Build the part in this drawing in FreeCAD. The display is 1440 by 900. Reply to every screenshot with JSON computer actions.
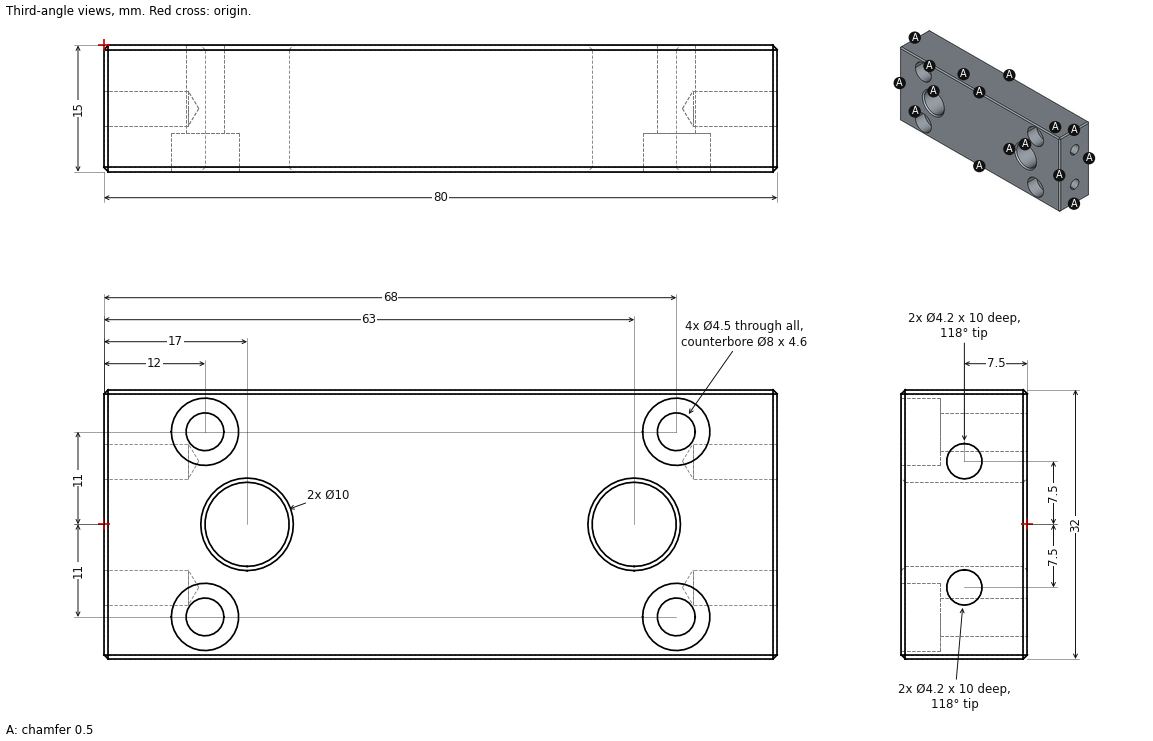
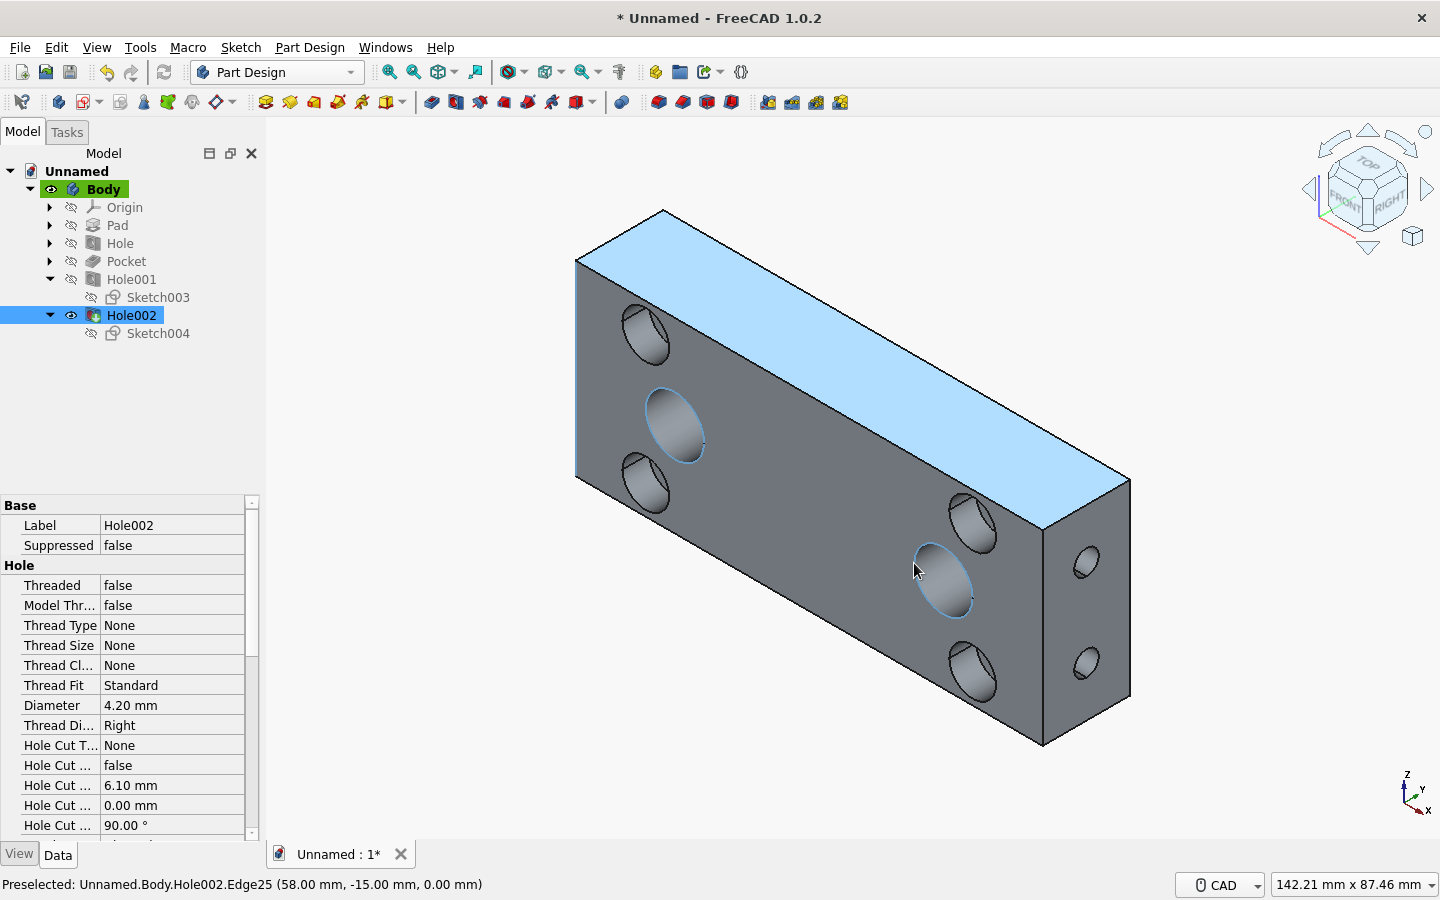
{"action": "left_click", "coordinate": [1043, 637], "text": "ctrl"}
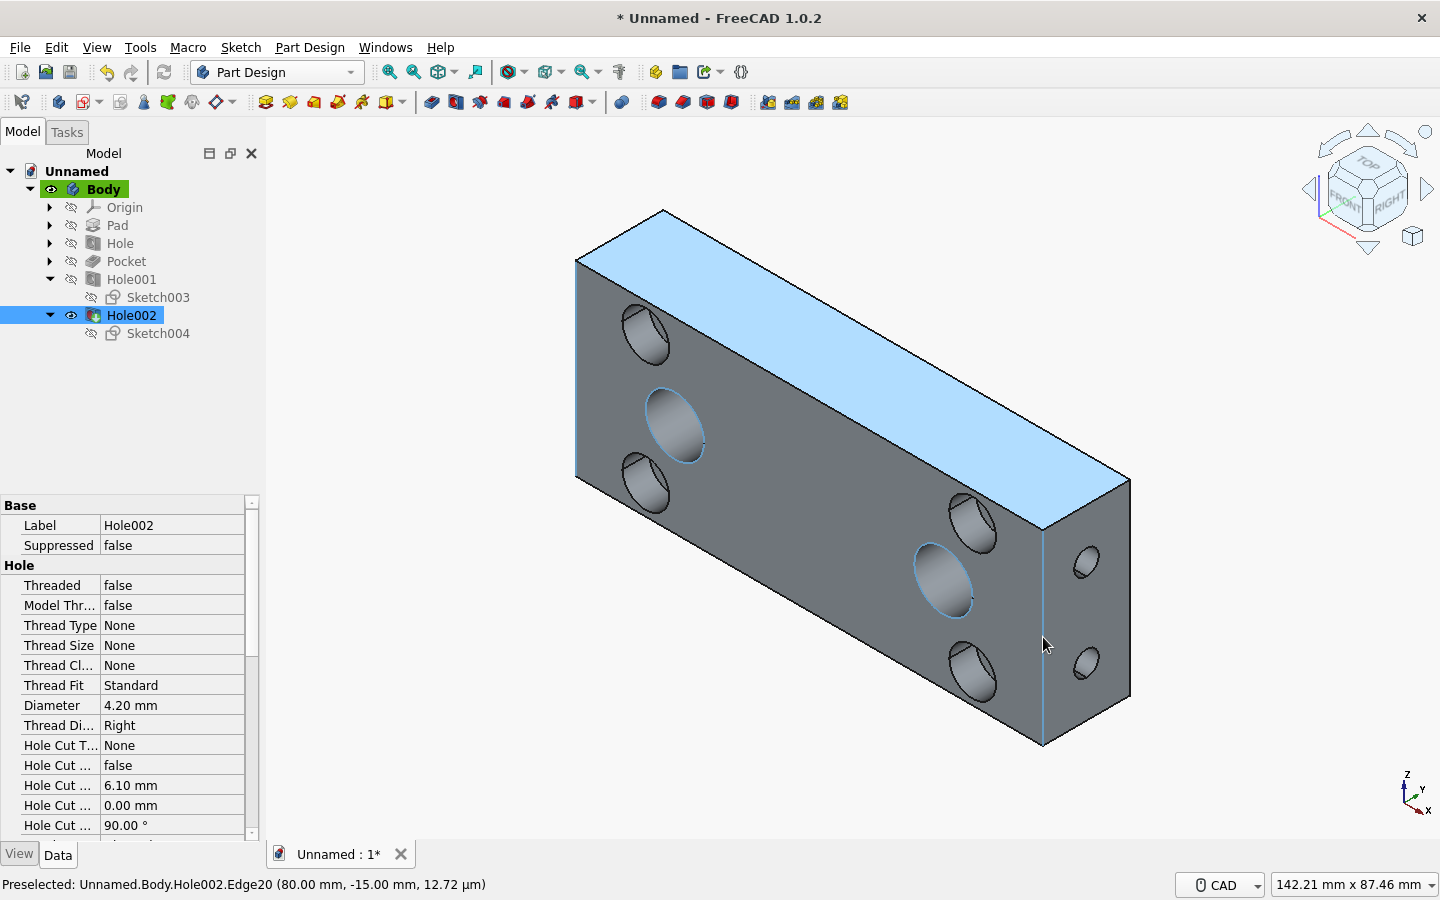
{"action": "key", "text": "2"}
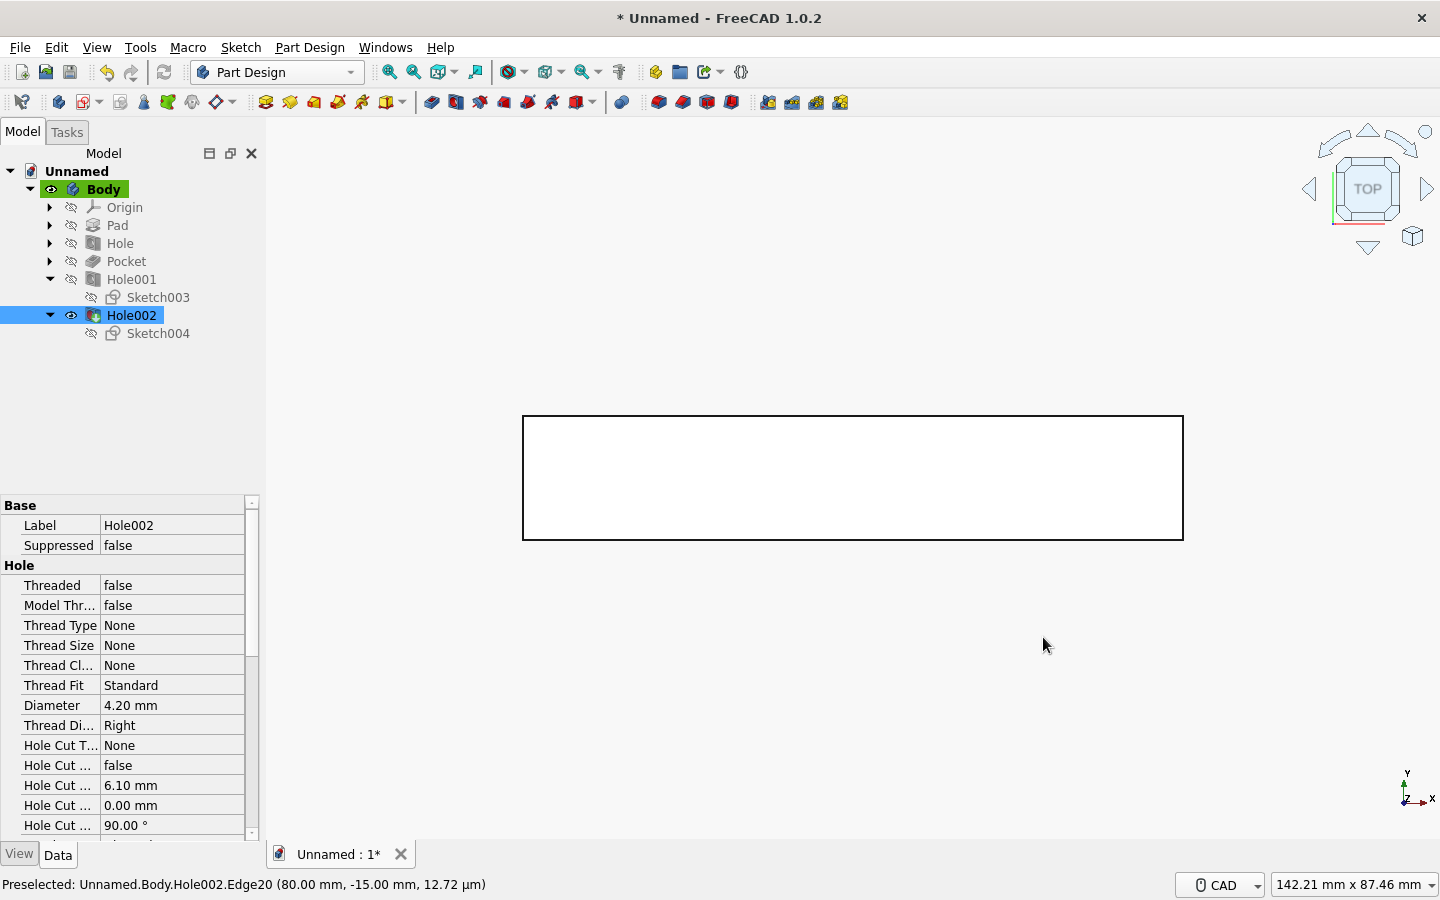
{"action": "key", "text": "1"}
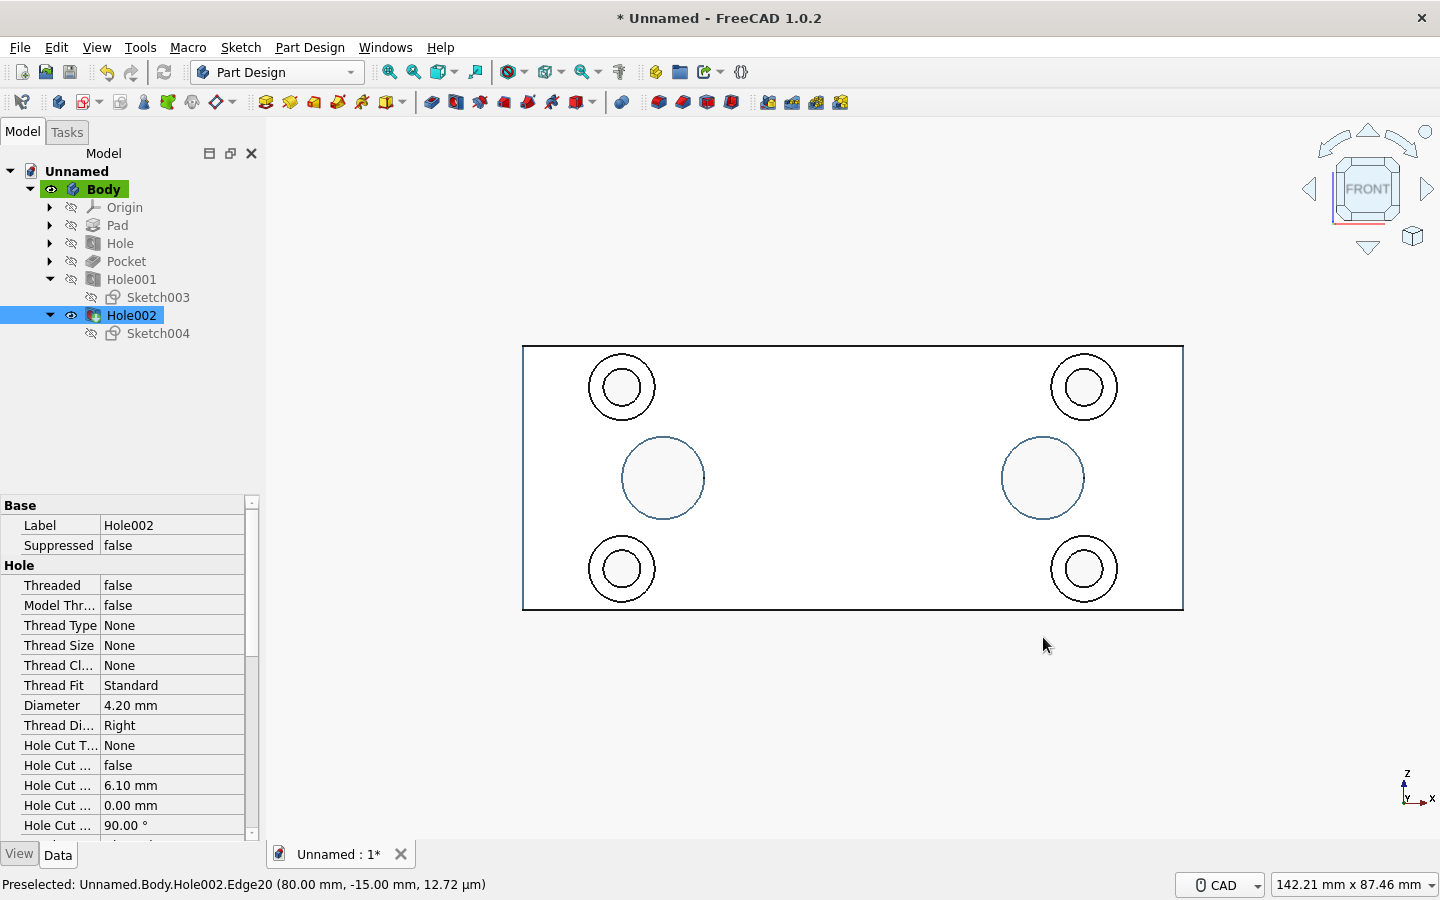
{"action": "key", "text": "3"}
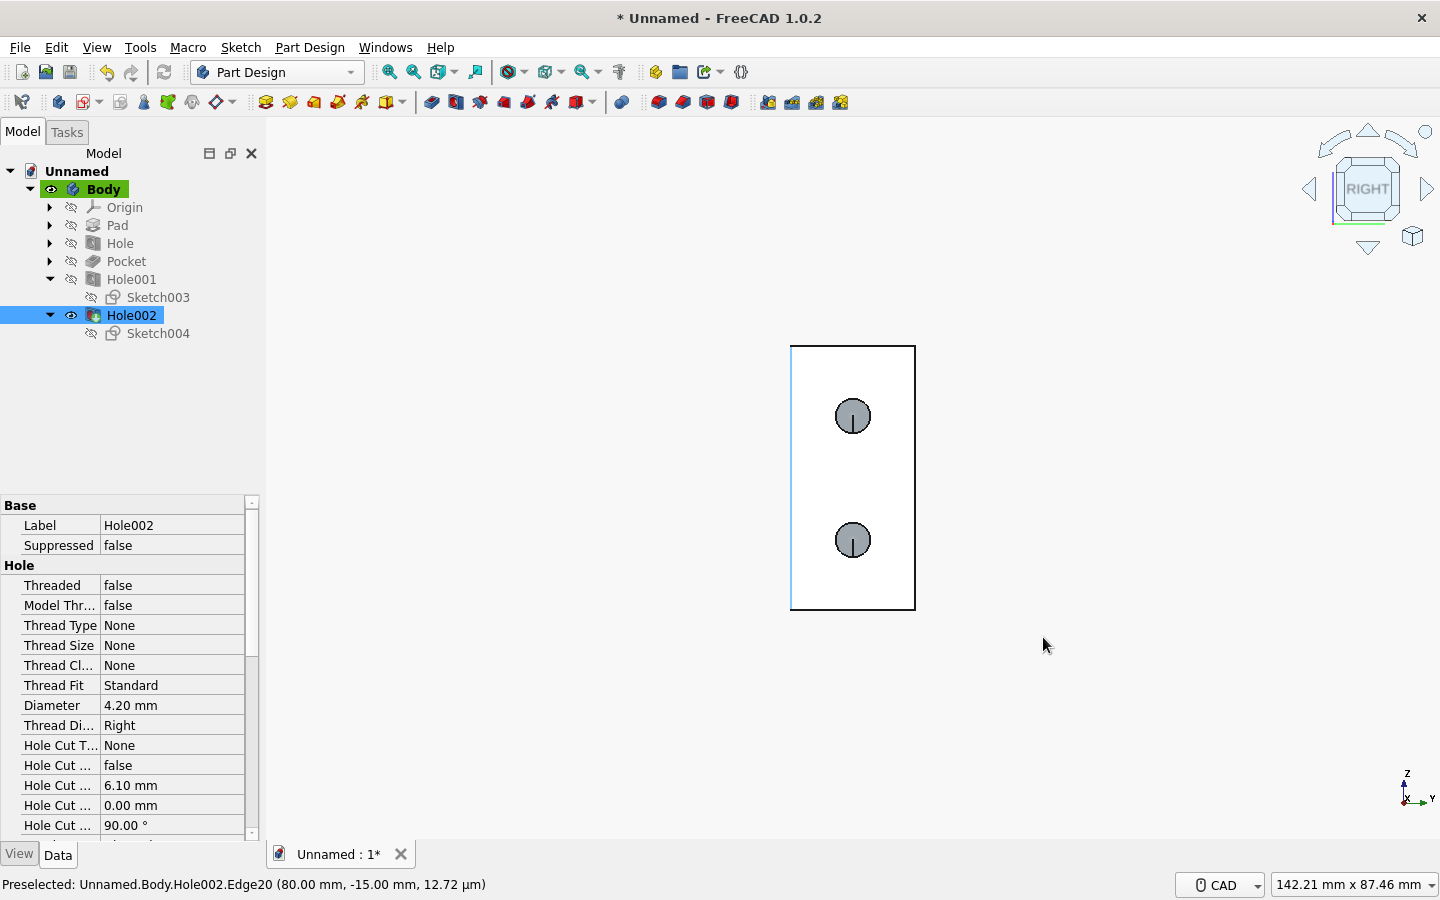
{"action": "left_click", "coordinate": [390, 72]}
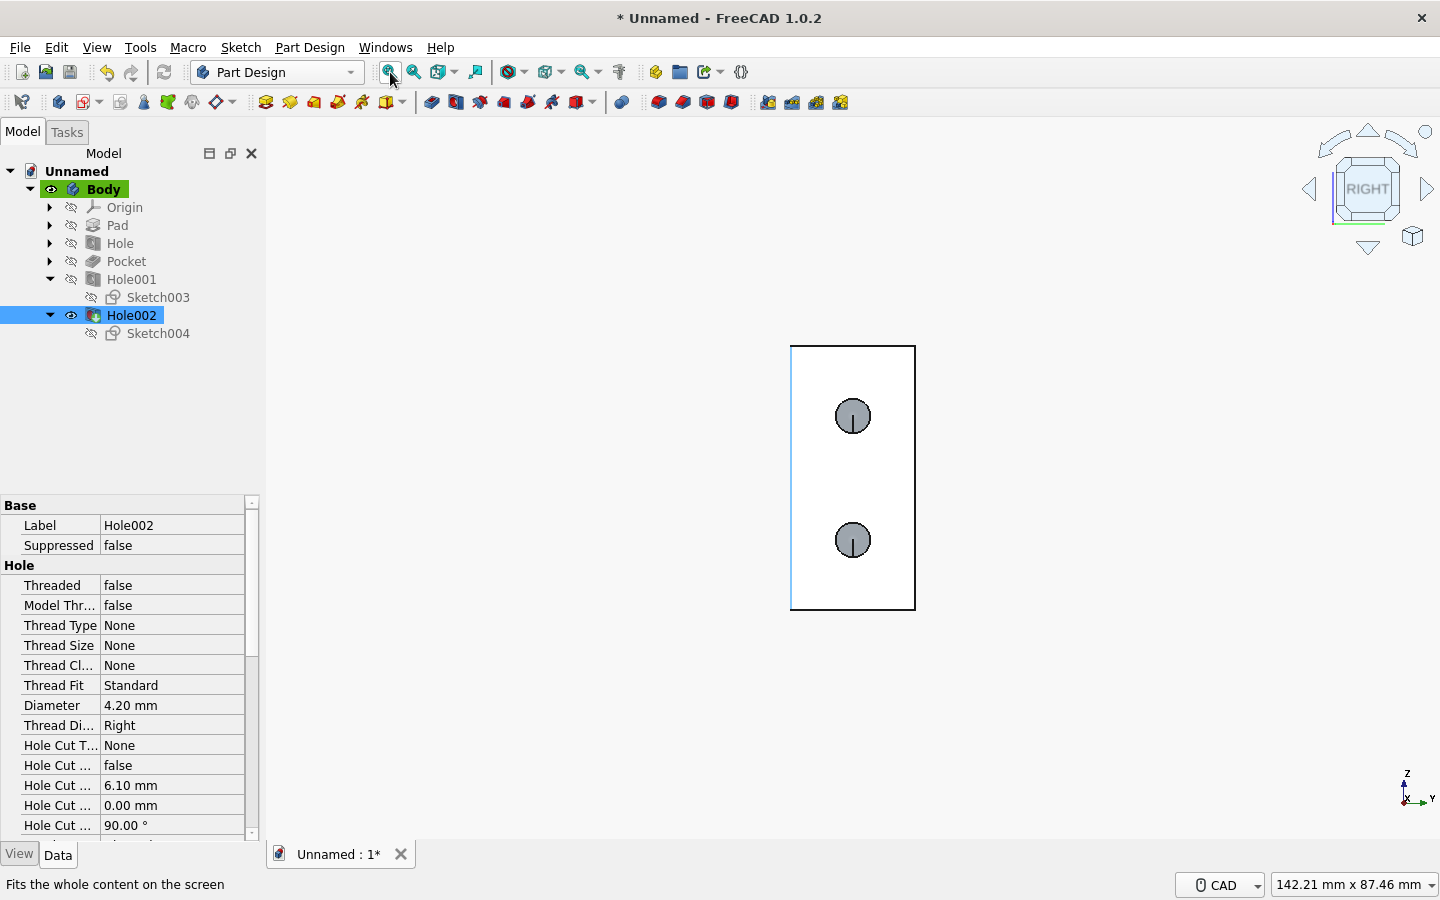
{"action": "left_click", "coordinate": [915, 477], "text": "ctrl"}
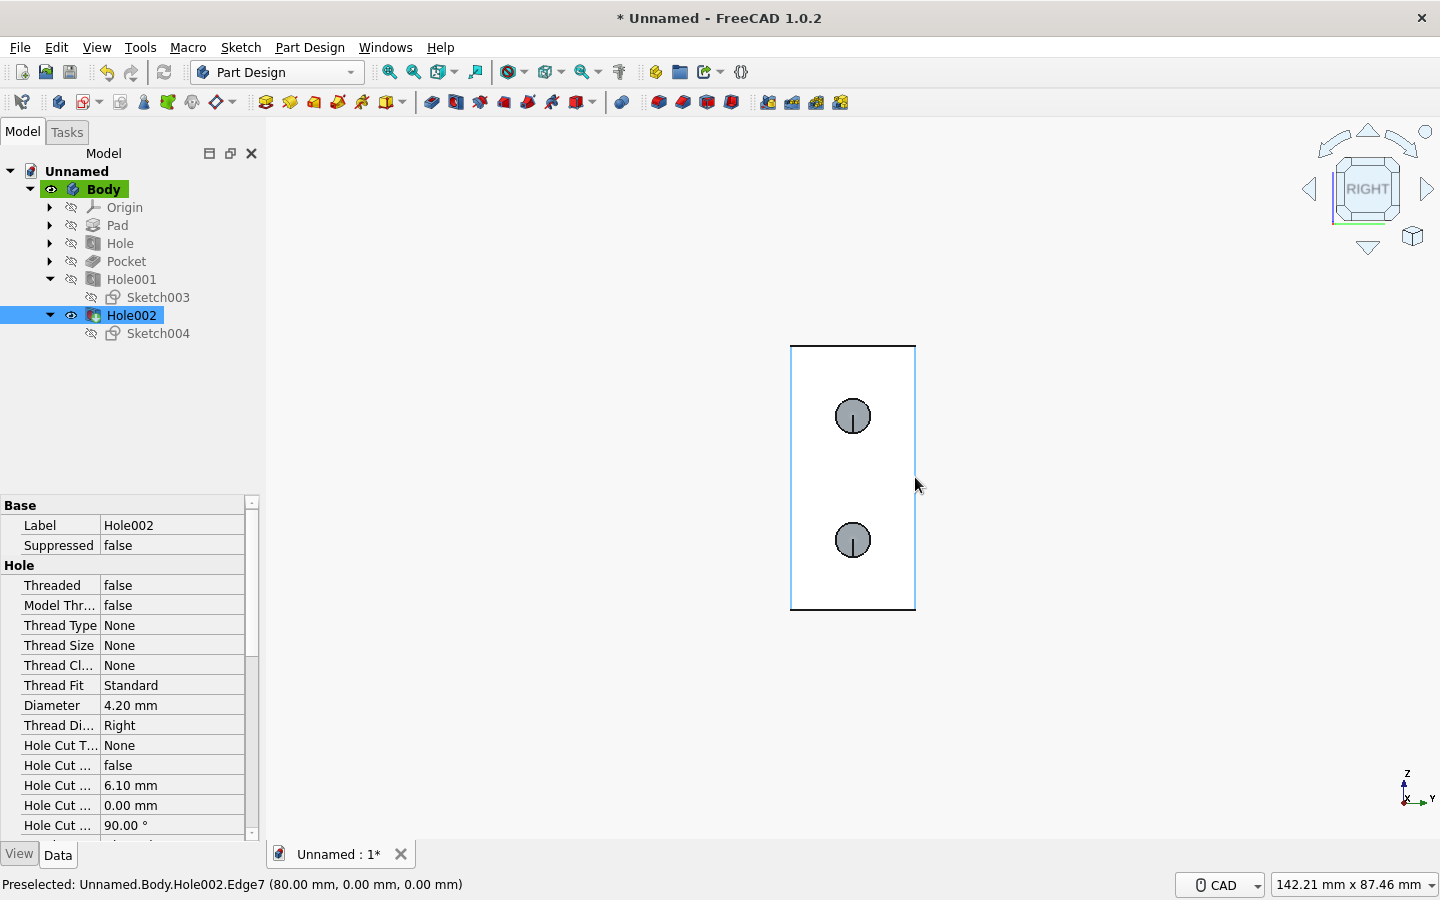
{"action": "key", "text": "5"}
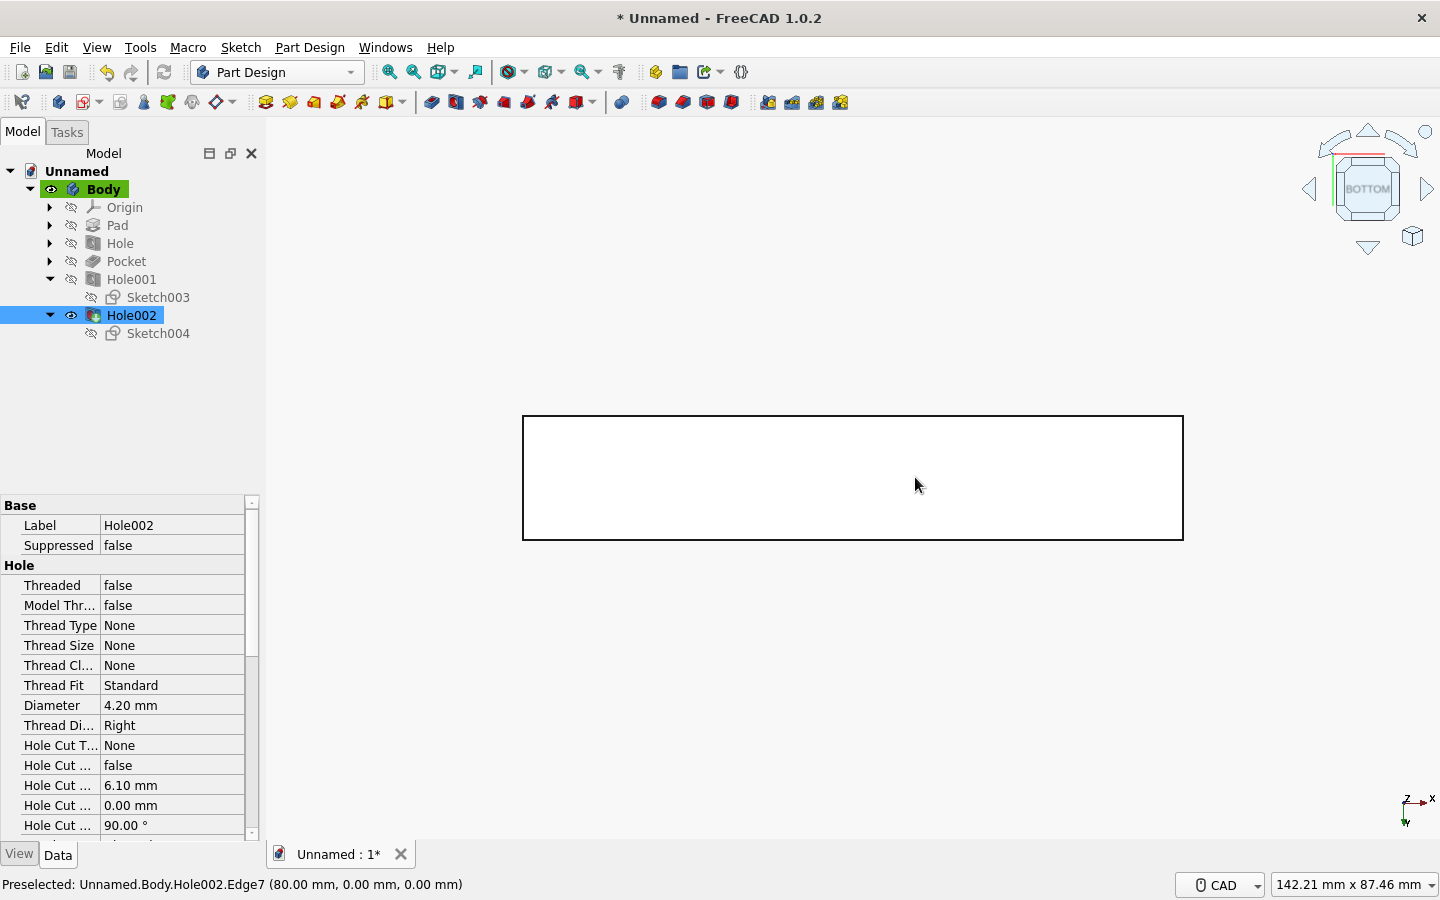
{"action": "left_click", "coordinate": [1042, 477], "text": "ctrl"}